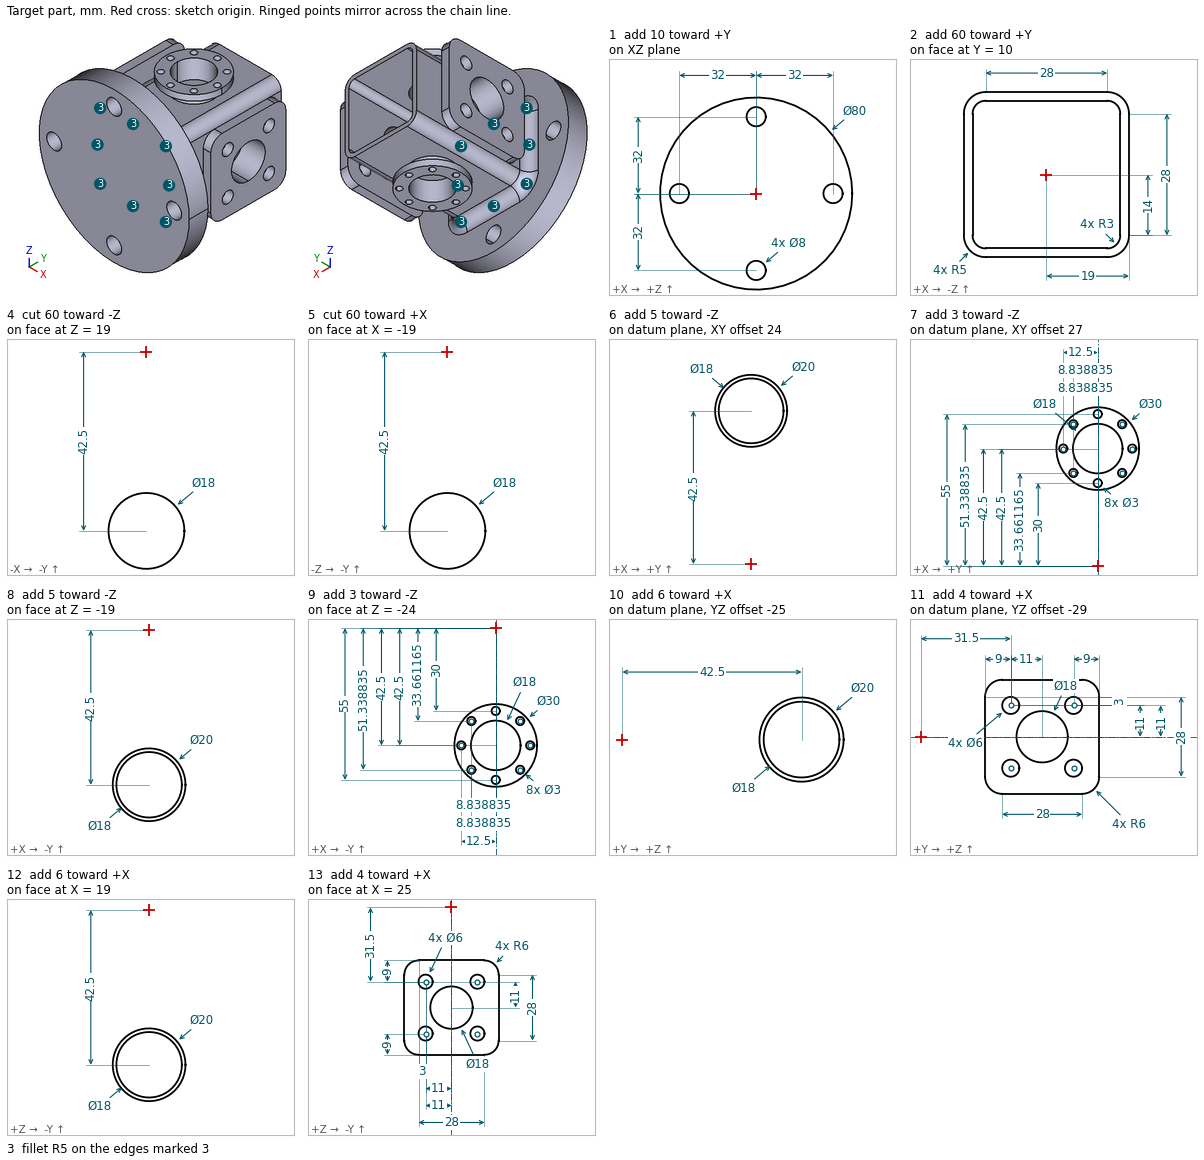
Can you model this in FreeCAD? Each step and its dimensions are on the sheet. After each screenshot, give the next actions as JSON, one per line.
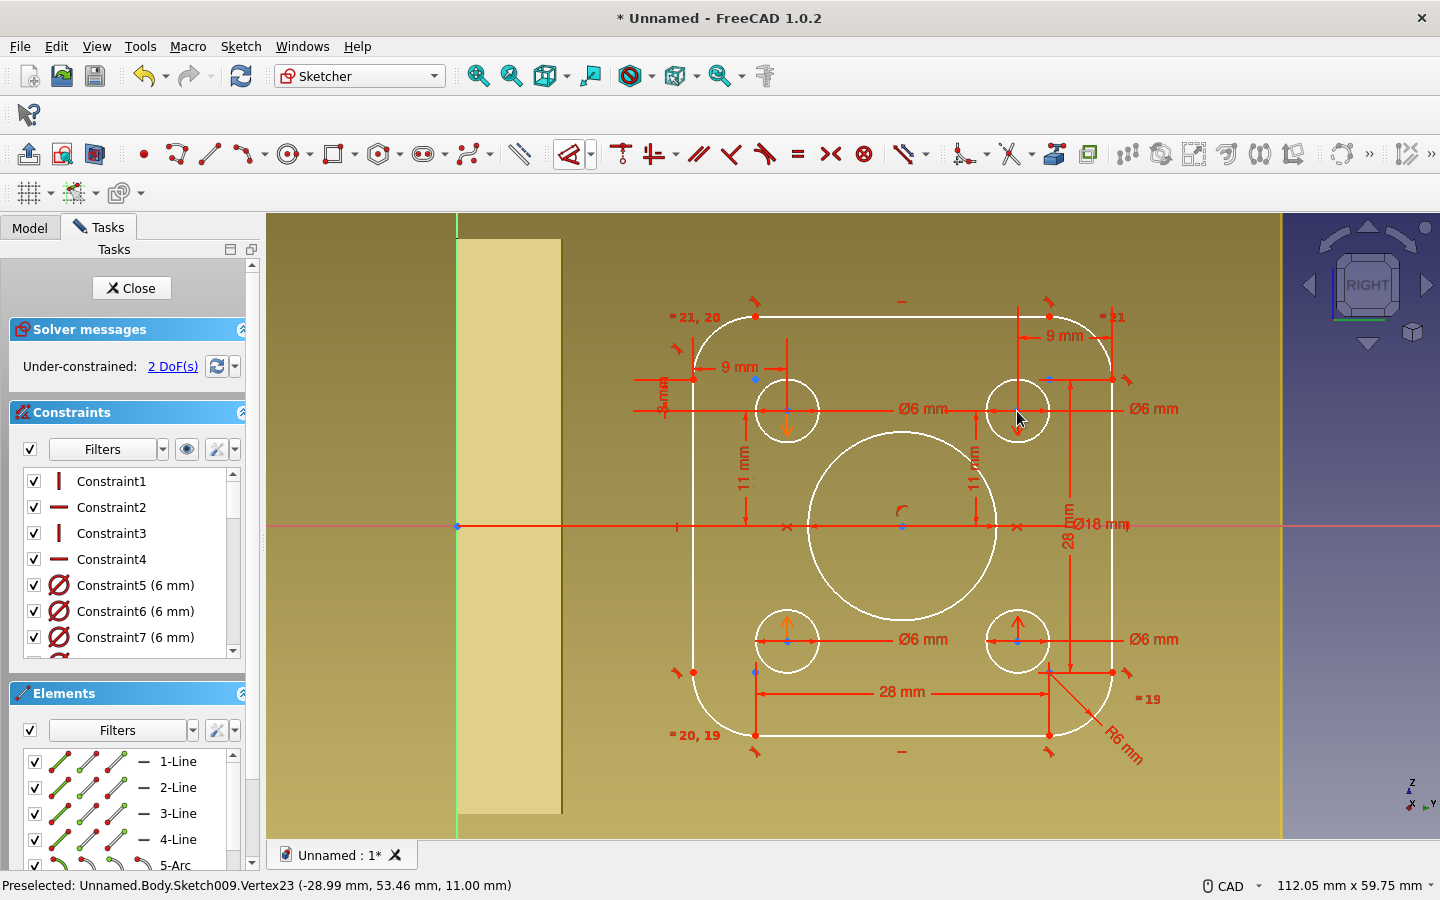
{"action": "left_click", "coordinate": [787, 411]}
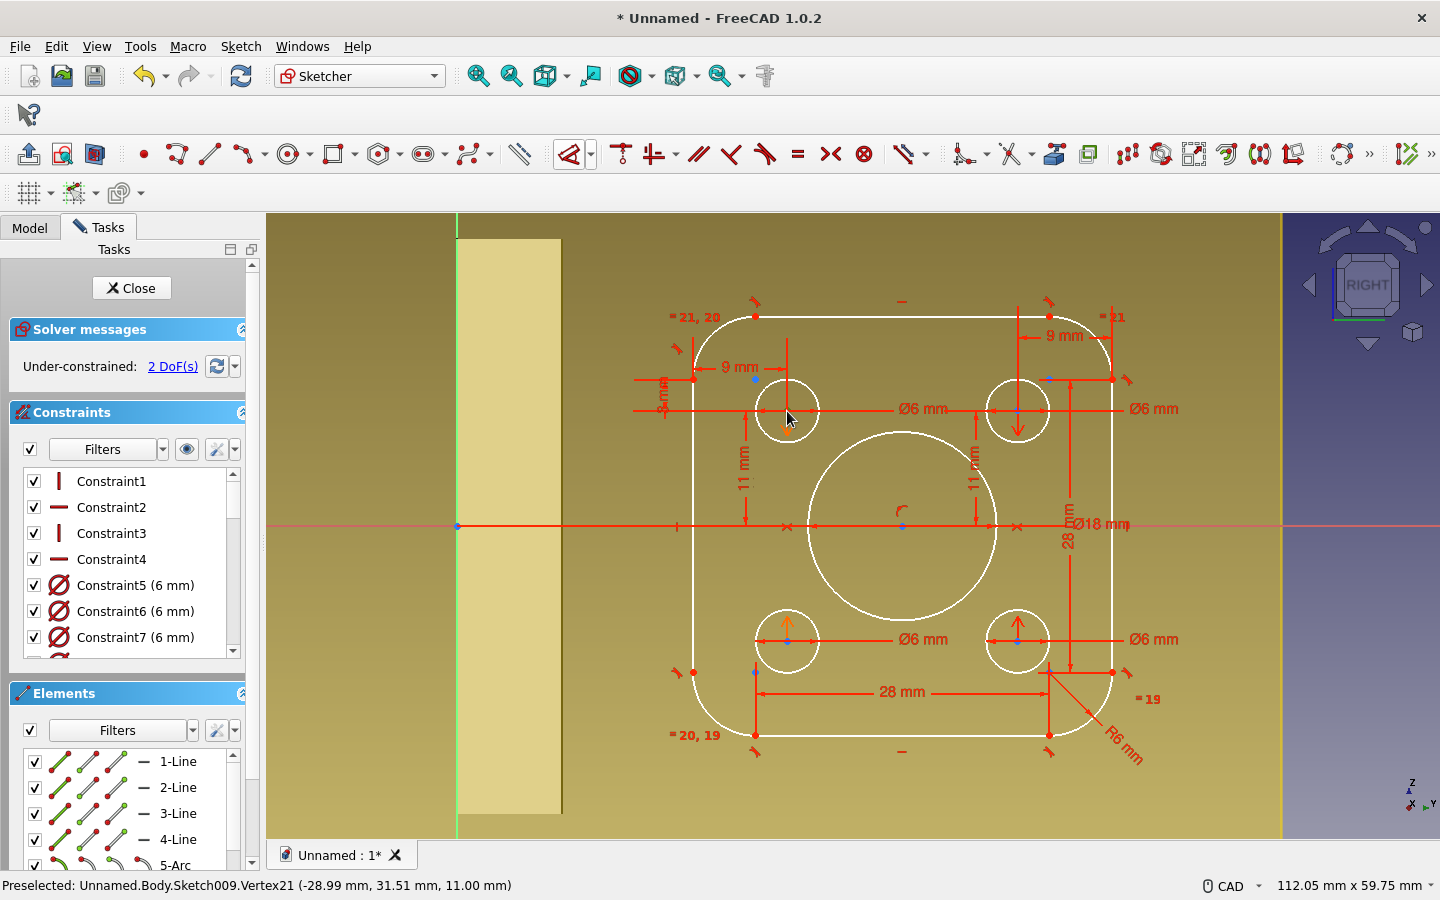
{"action": "left_click", "coordinate": [902, 526]}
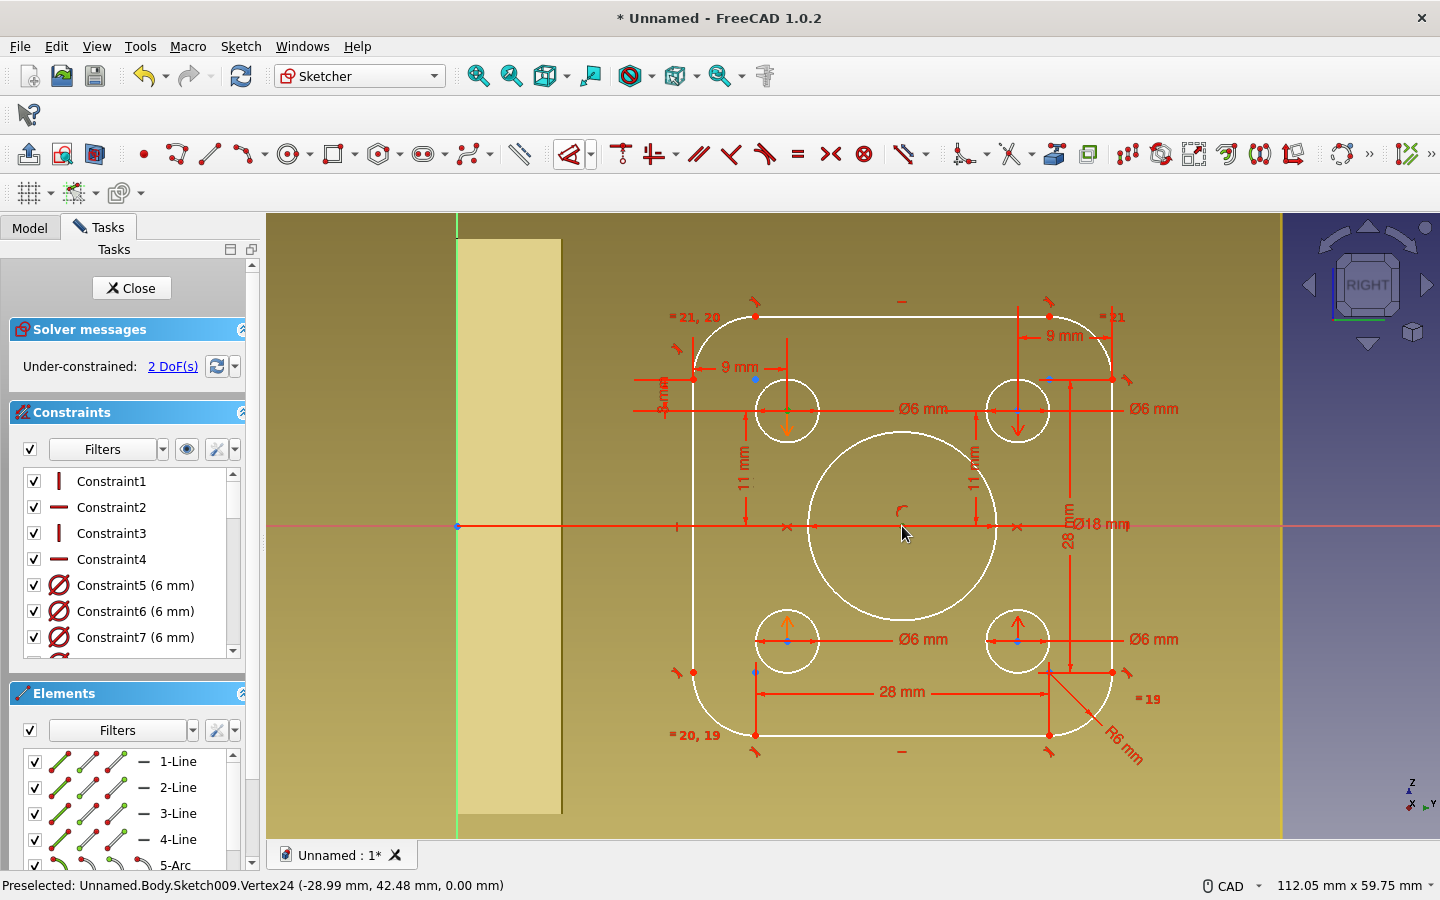
{"action": "key", "text": "l"}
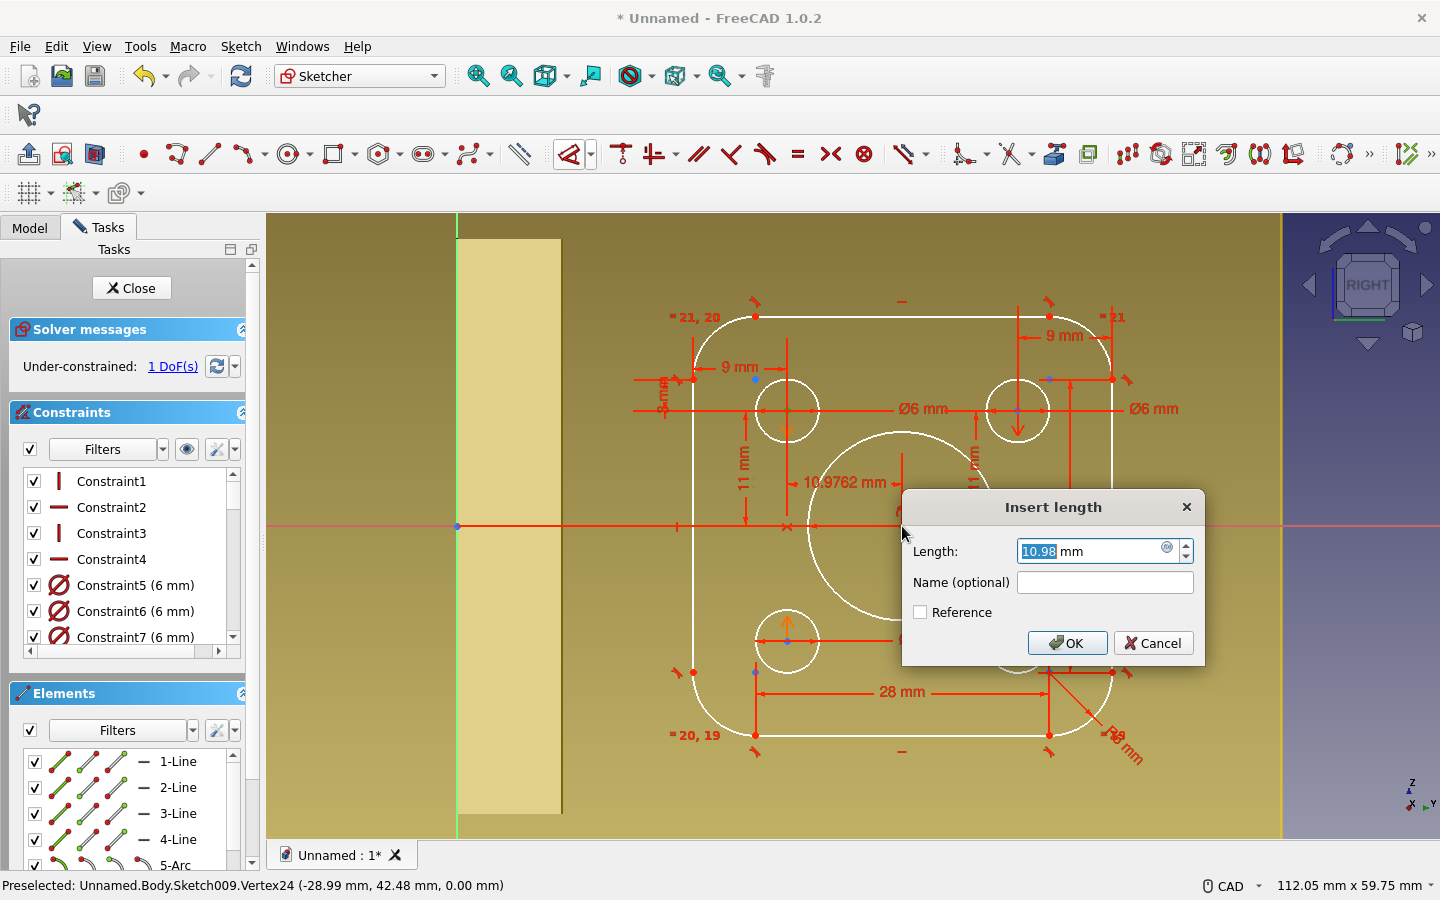
{"action": "type", "text": "11"}
{"action": "key", "text": "Return"}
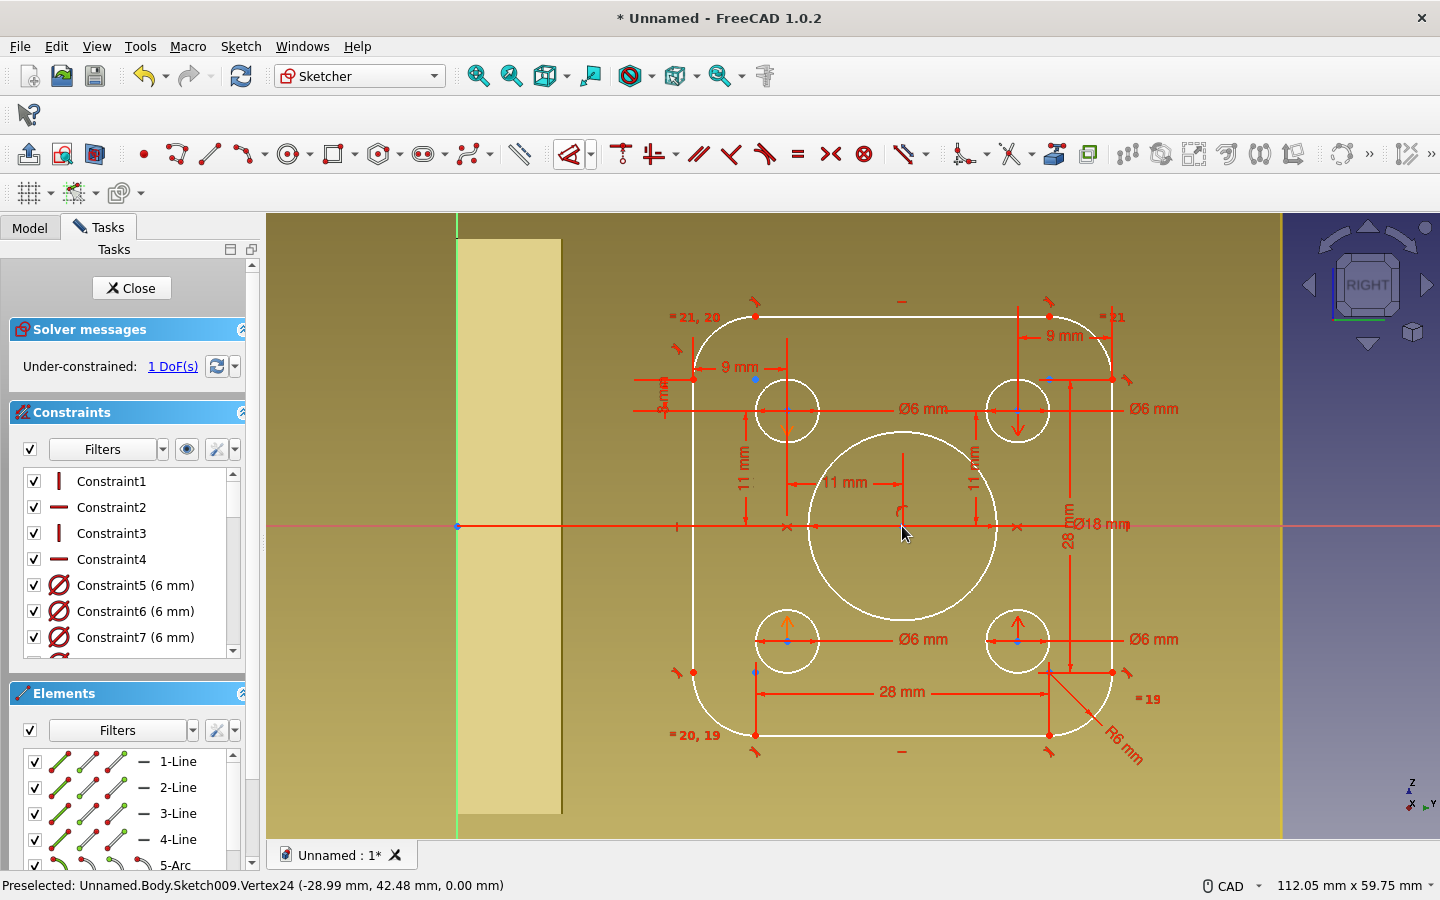
{"action": "left_click", "coordinate": [787, 411]}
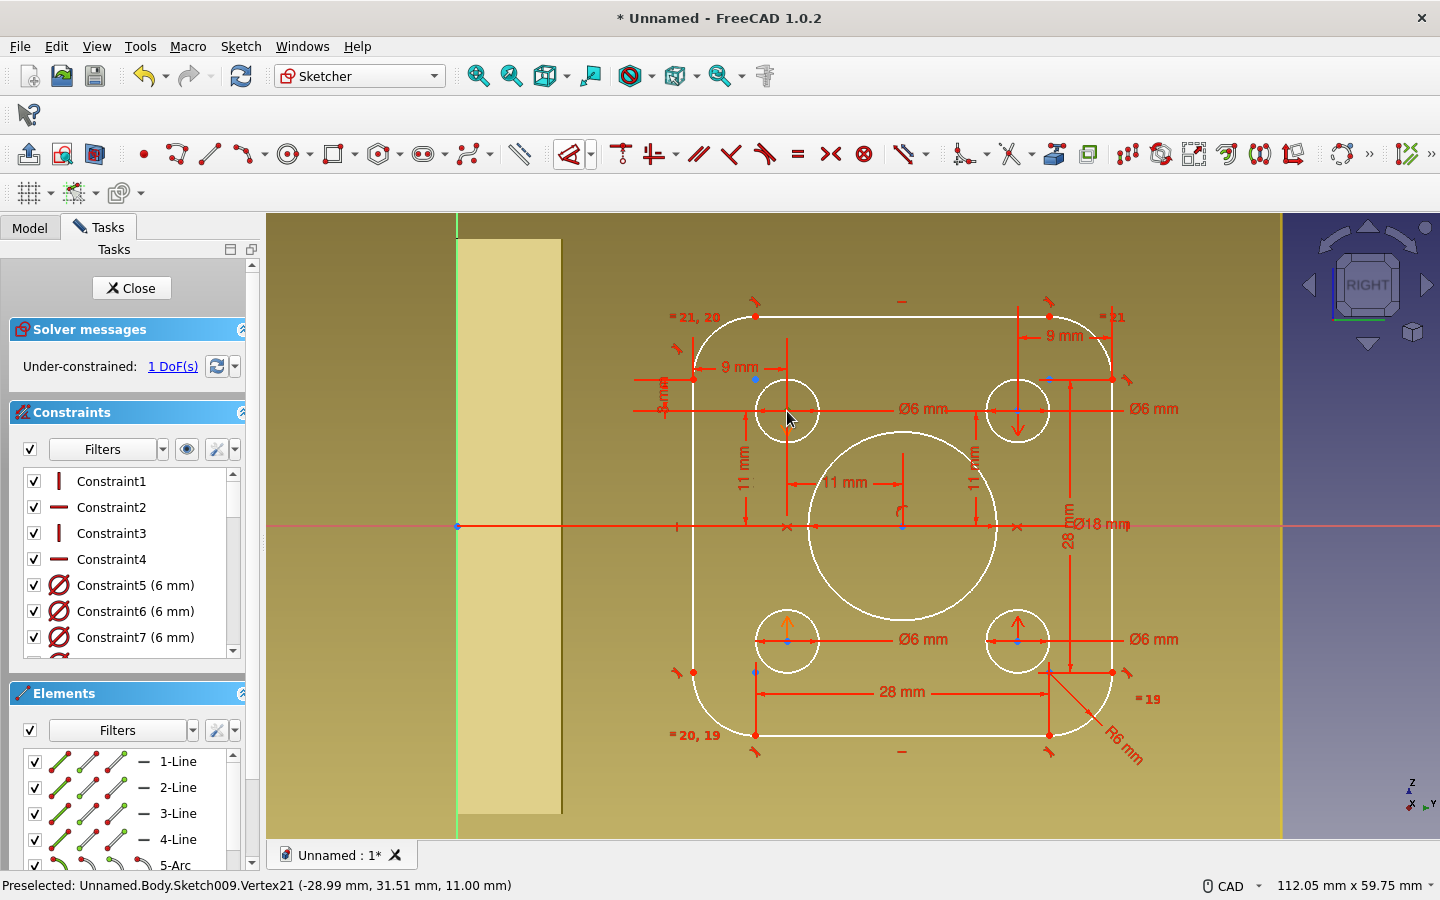
{"action": "key", "text": "l"}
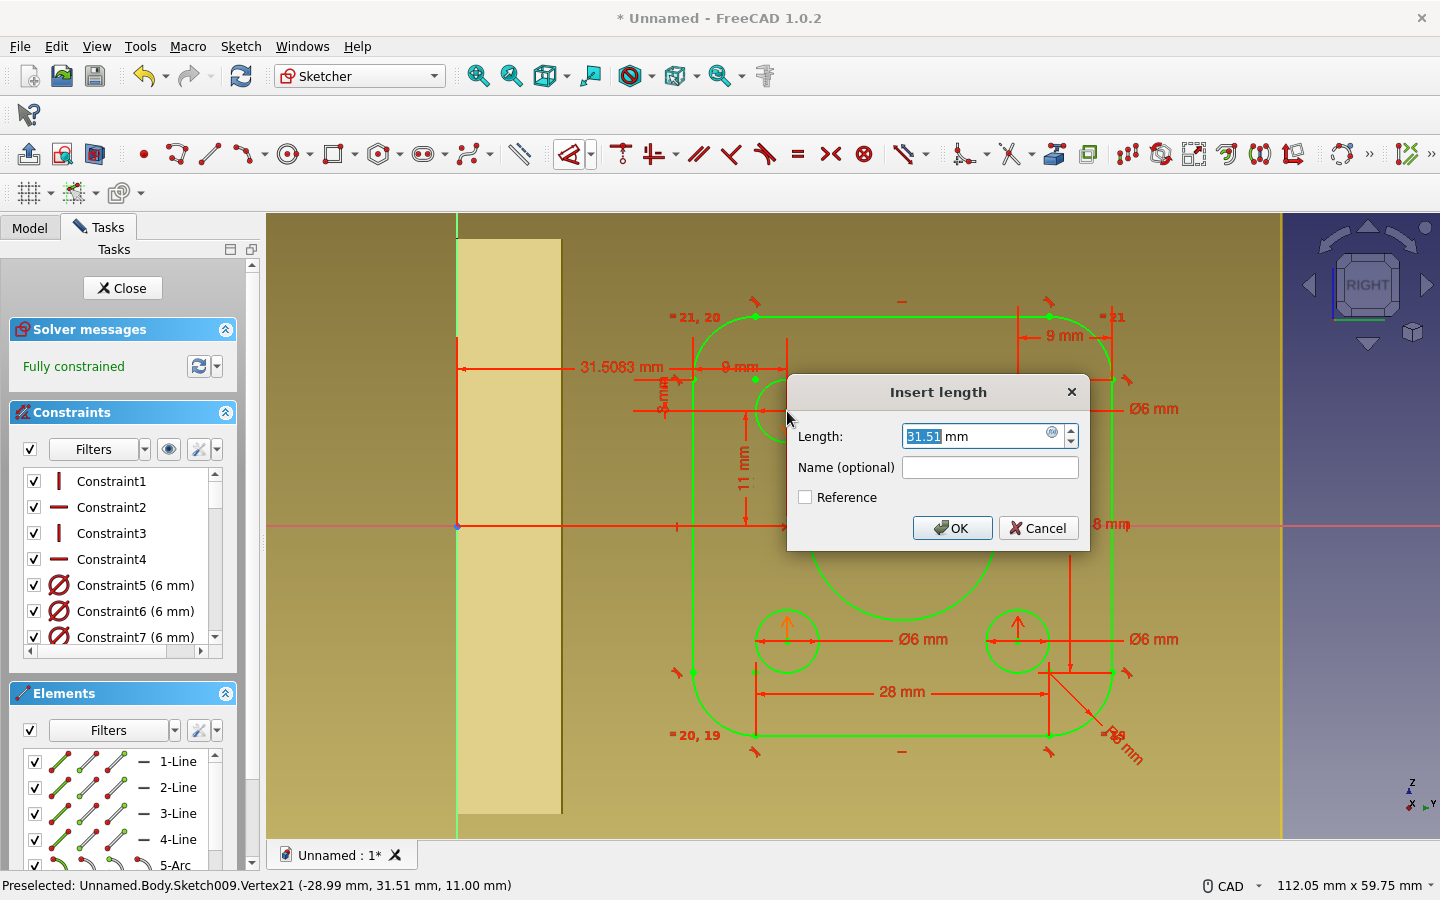
{"action": "type", "text": "31.5"}
{"action": "key", "text": "Return"}